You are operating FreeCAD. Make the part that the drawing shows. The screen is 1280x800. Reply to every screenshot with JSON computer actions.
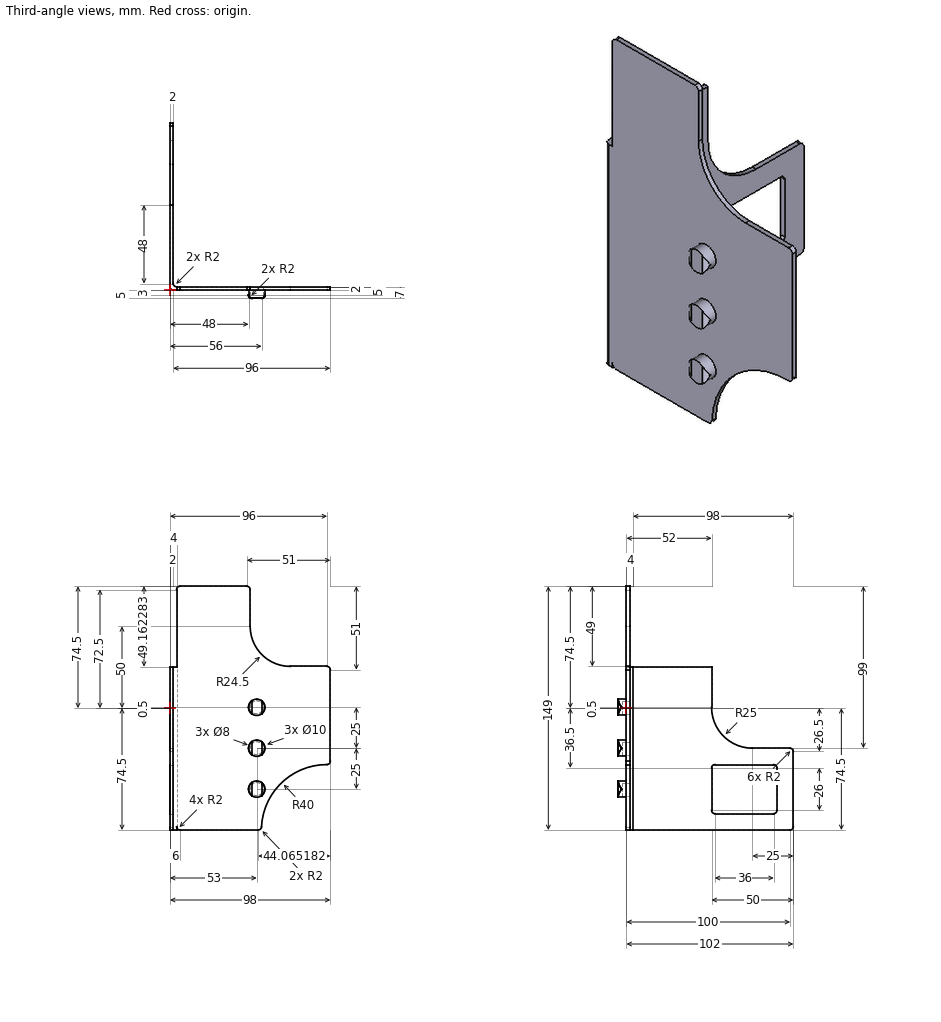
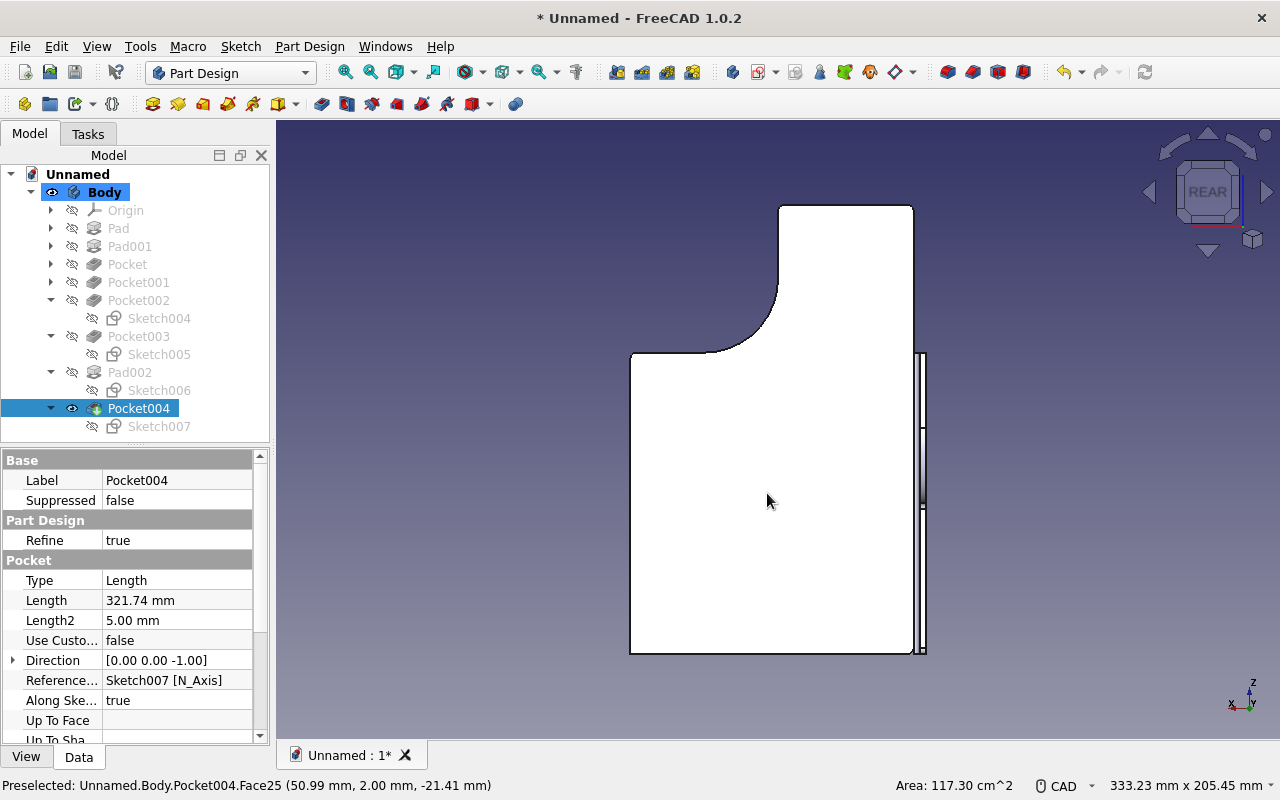
{"action": "left_click", "coordinate": [758, 72]}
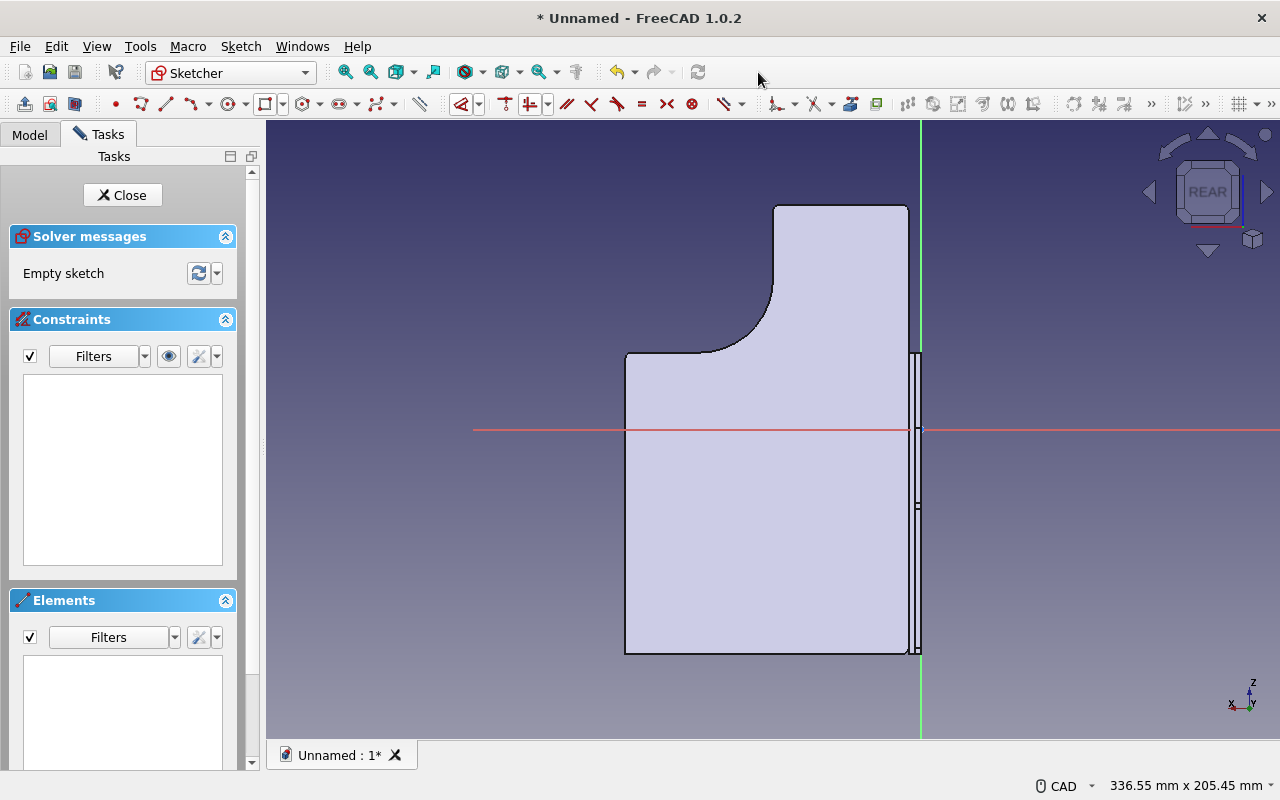
{"action": "scroll", "coordinate": [941, 564], "scroll_direction": "up", "scroll_amount": 4}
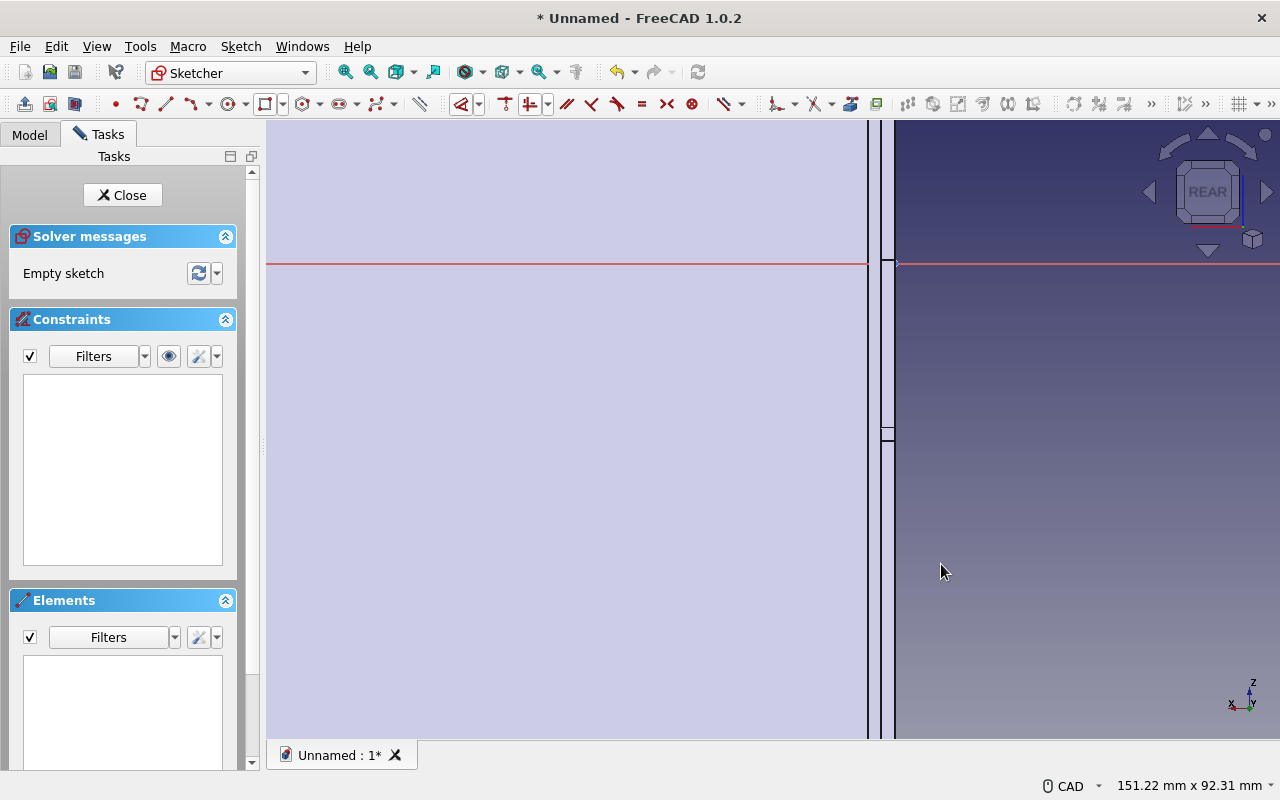
{"action": "key", "text": "g c"}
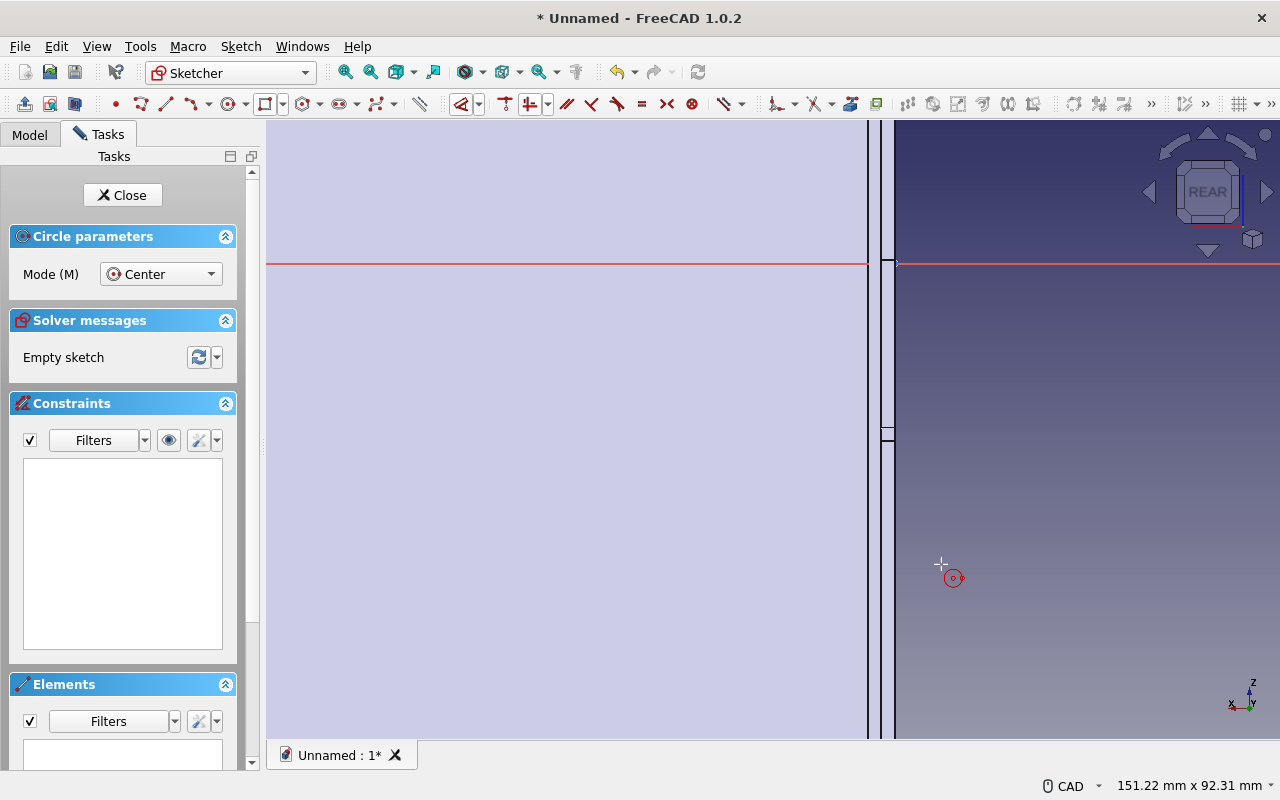
{"action": "left_click", "coordinate": [539, 428]}
{"action": "mouse_move", "coordinate": [558, 409]}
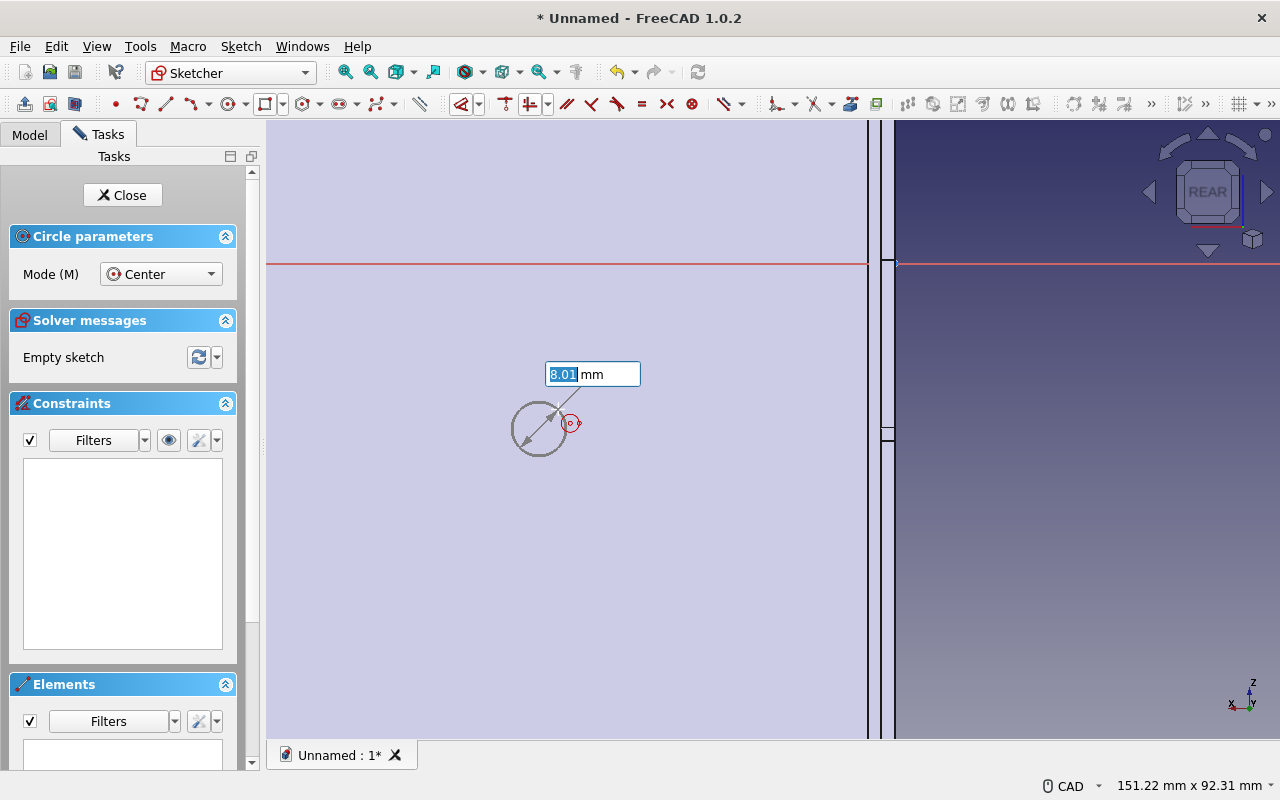
{"action": "type", "text": "8"}
{"action": "key", "text": "Return"}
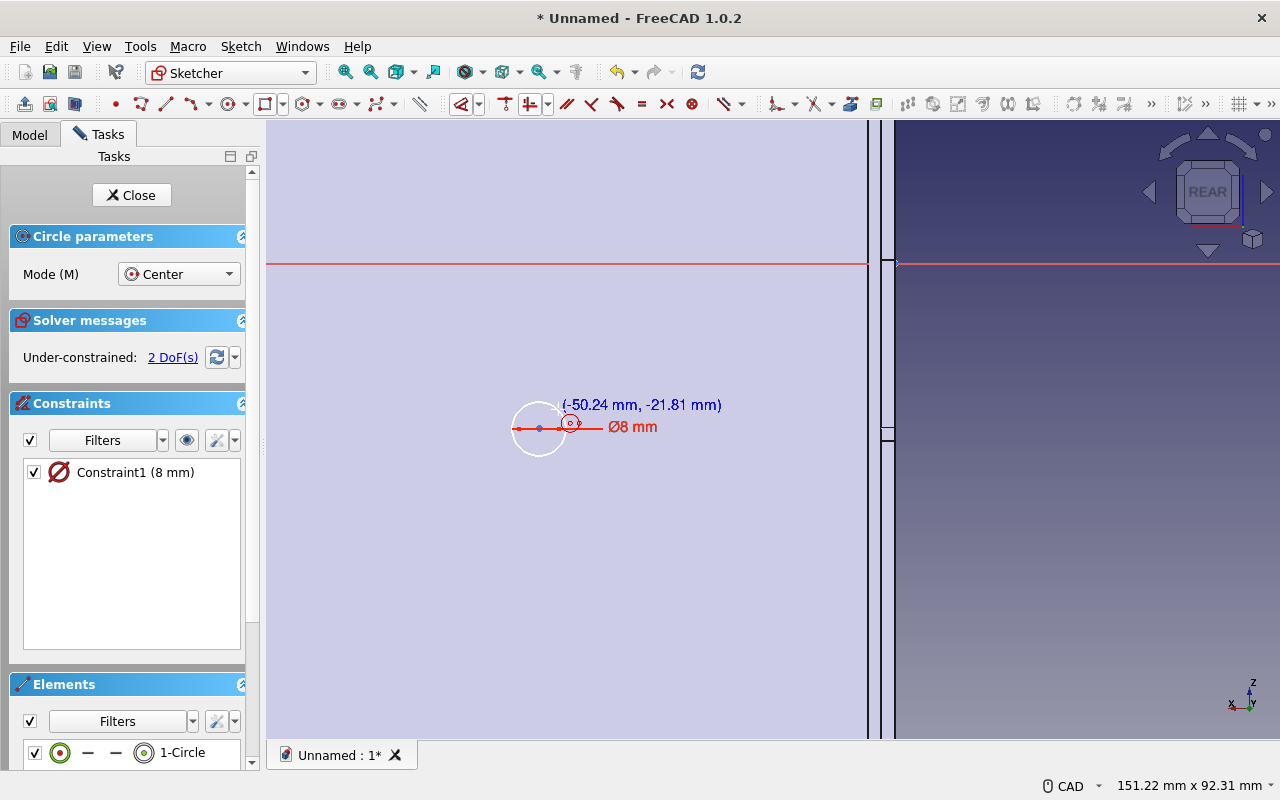
{"action": "left_click", "coordinate": [539, 596]}
{"action": "mouse_move", "coordinate": [558, 577]}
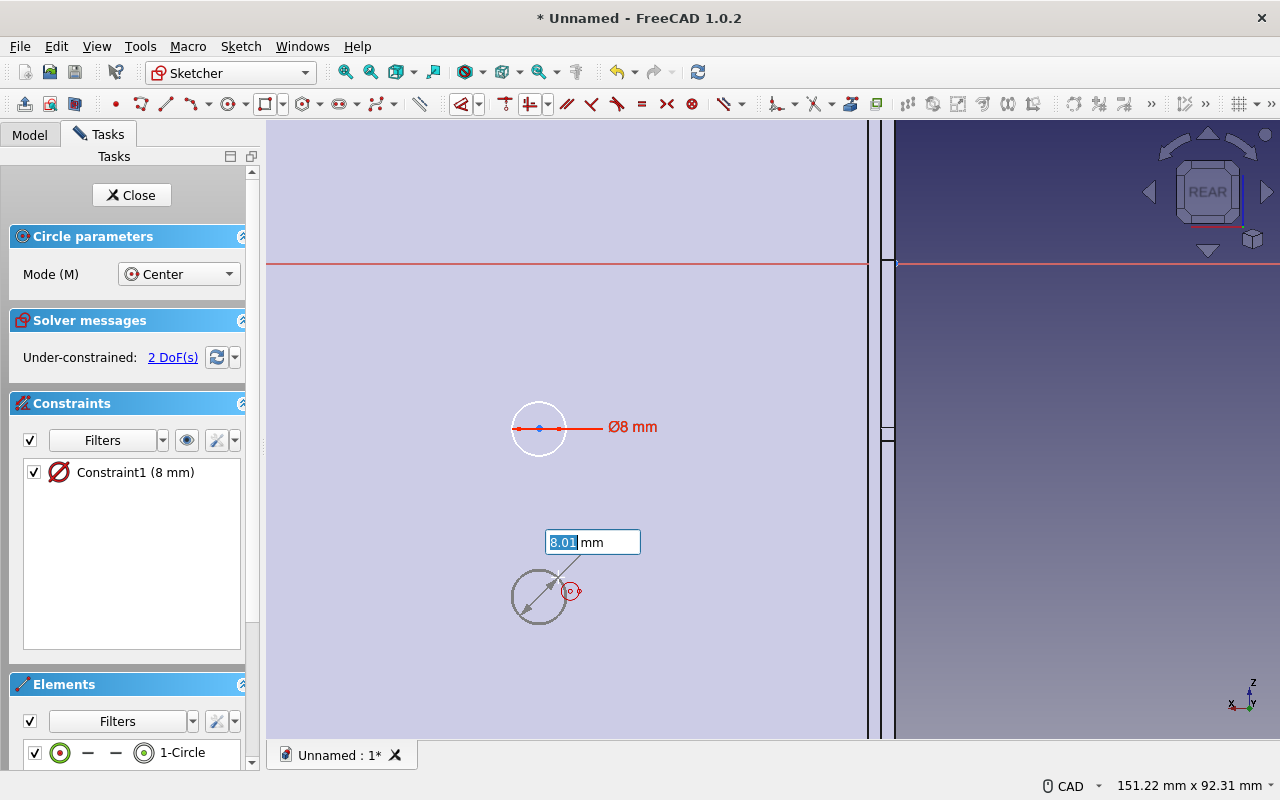
{"action": "type", "text": "8"}
{"action": "key", "text": "Return"}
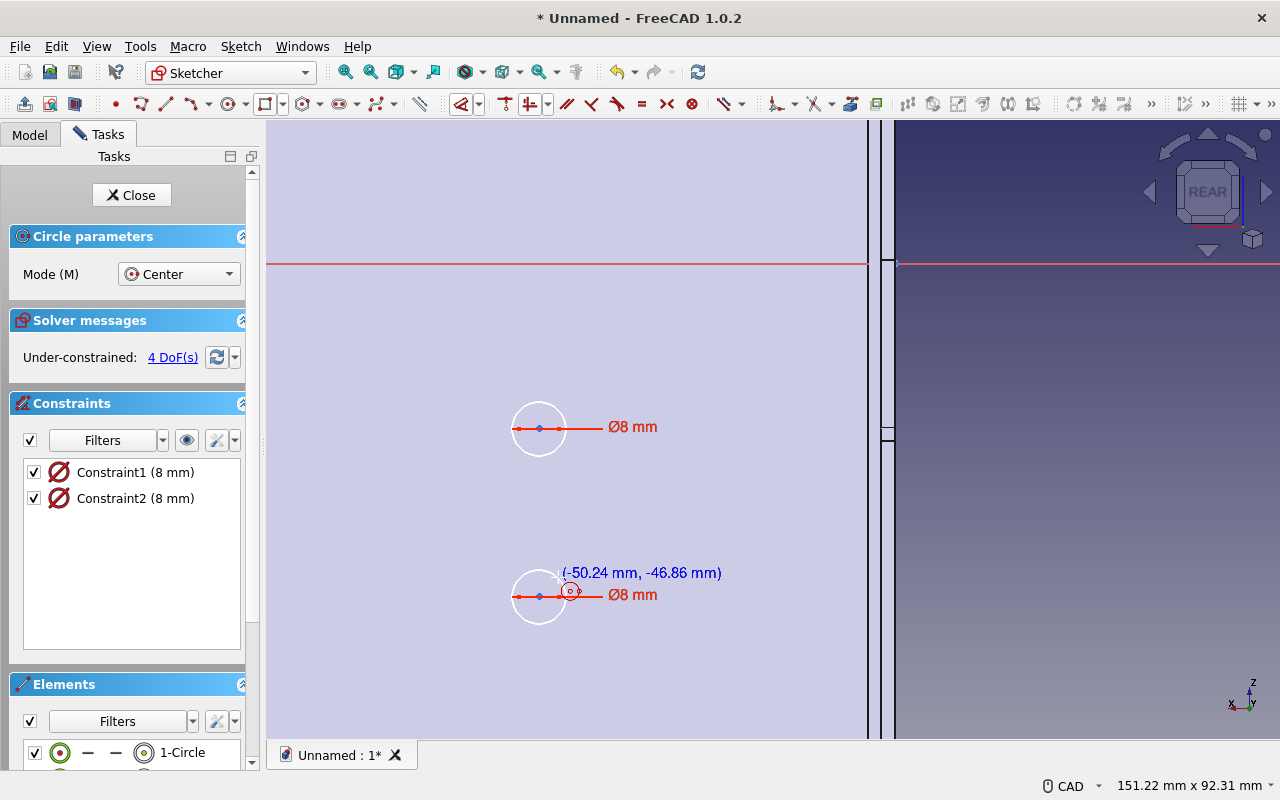
{"action": "scroll", "coordinate": [539, 260], "scroll_direction": "up", "scroll_amount": 8}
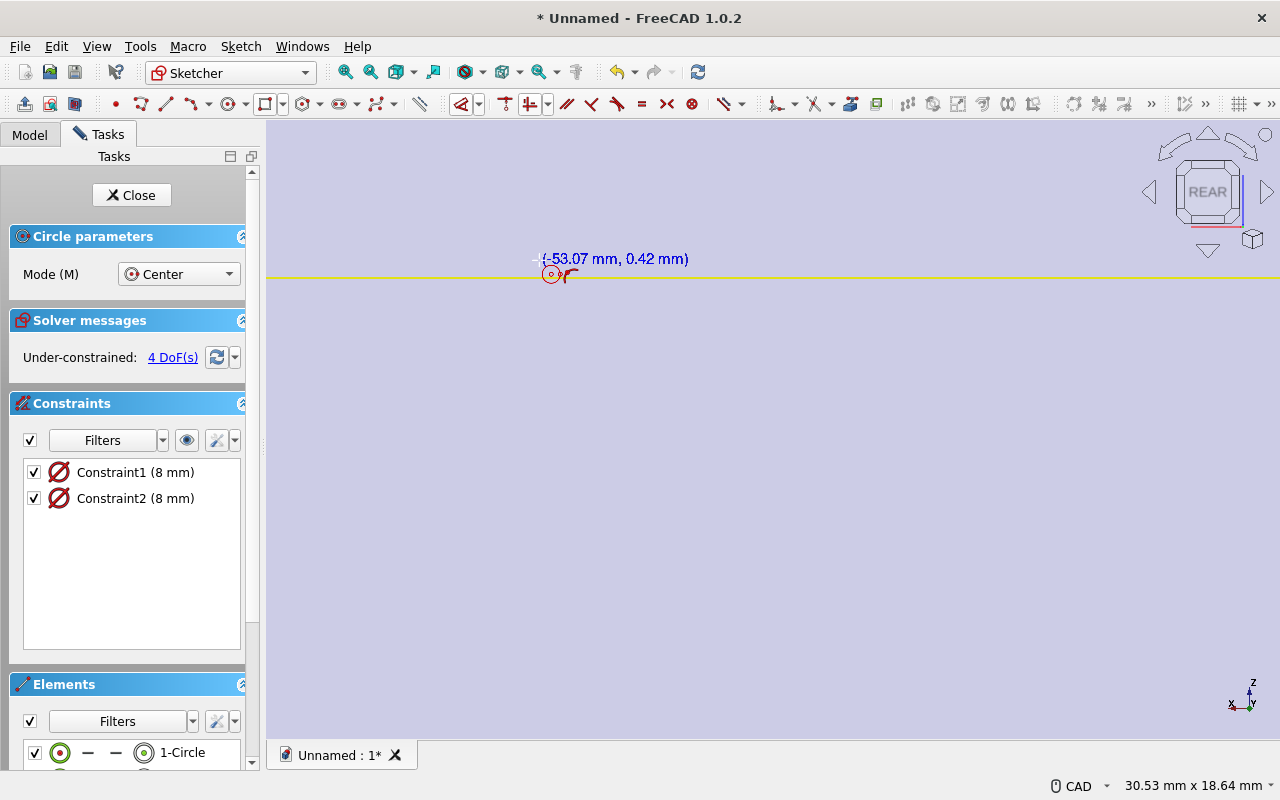
{"action": "left_click", "coordinate": [540, 261]}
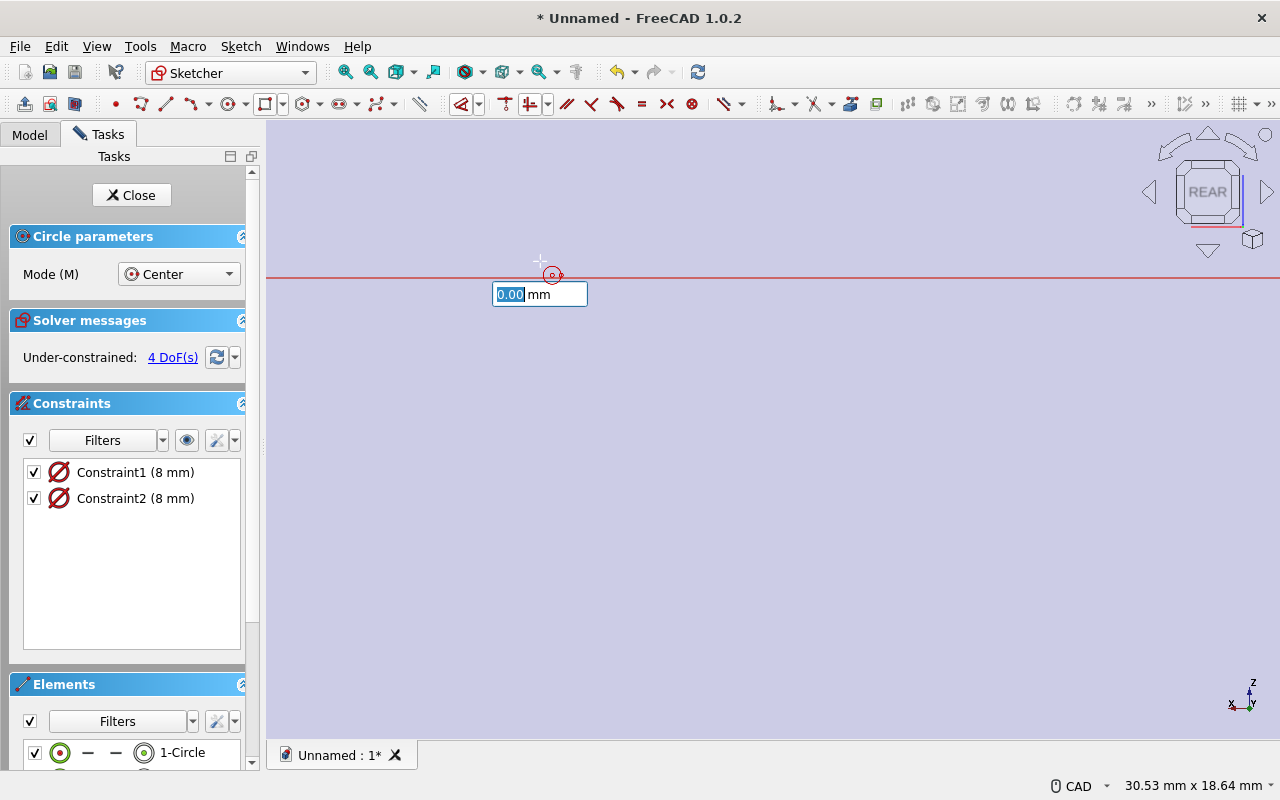
{"action": "scroll", "coordinate": [540, 262], "scroll_direction": "down", "scroll_amount": 8}
{"action": "mouse_move", "coordinate": [559, 243]}